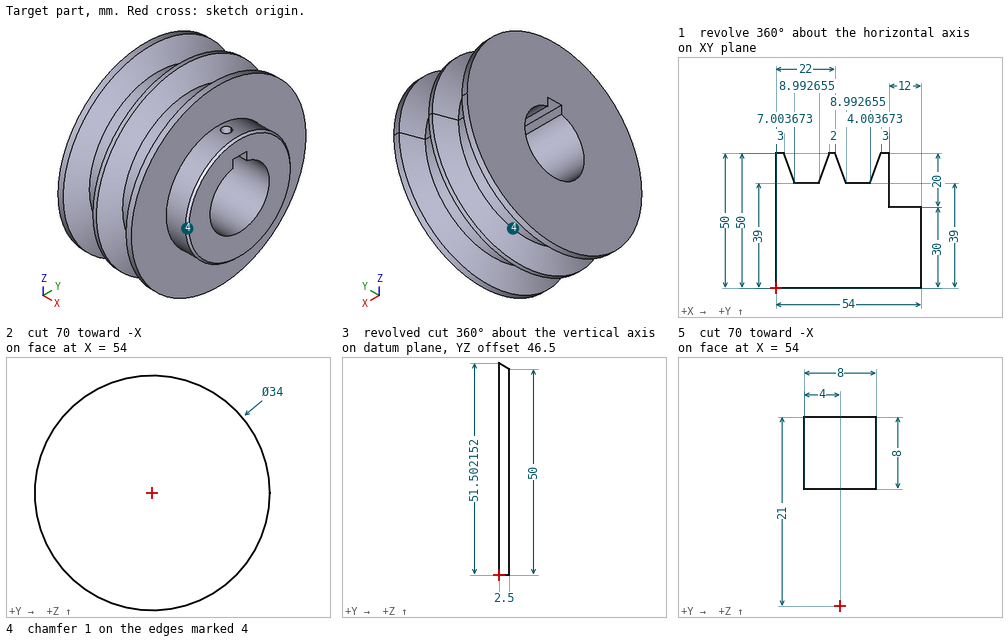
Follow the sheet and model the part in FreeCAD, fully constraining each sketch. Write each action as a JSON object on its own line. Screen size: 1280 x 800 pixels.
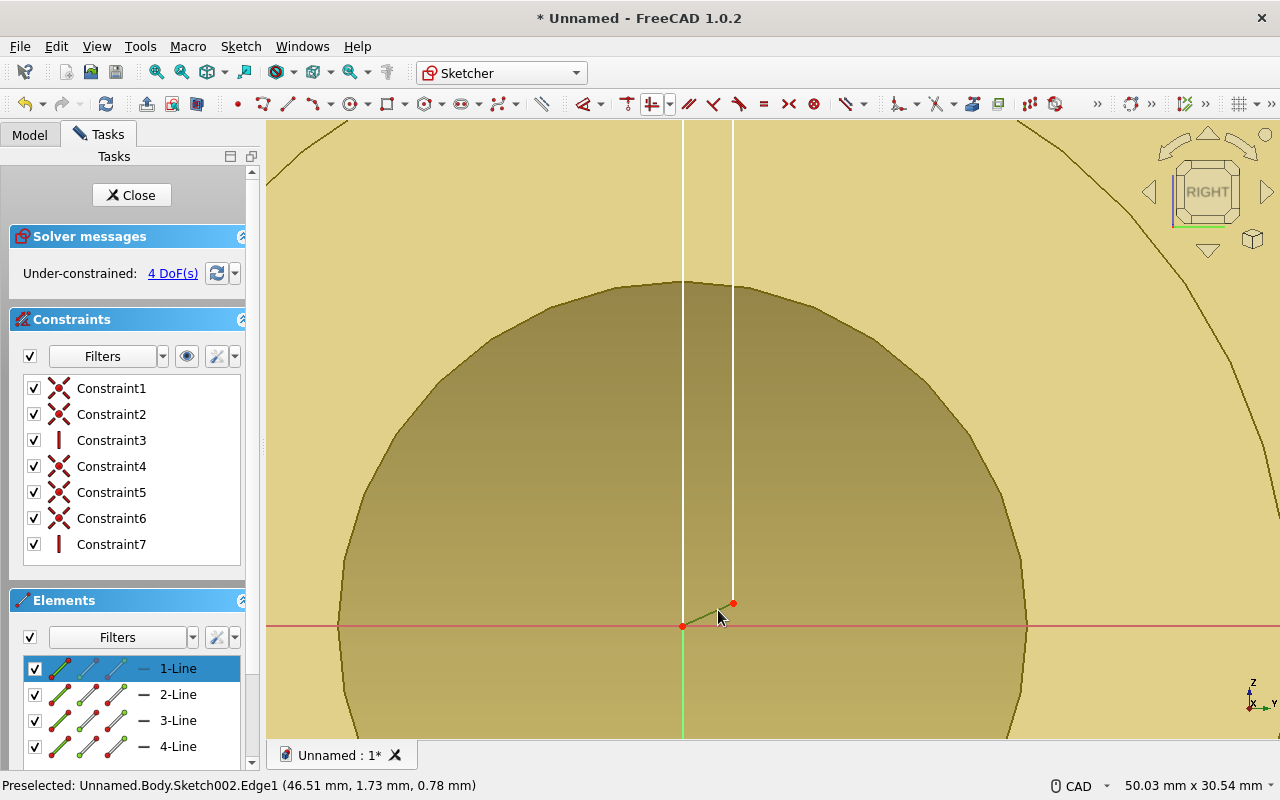
{"action": "key", "text": "h"}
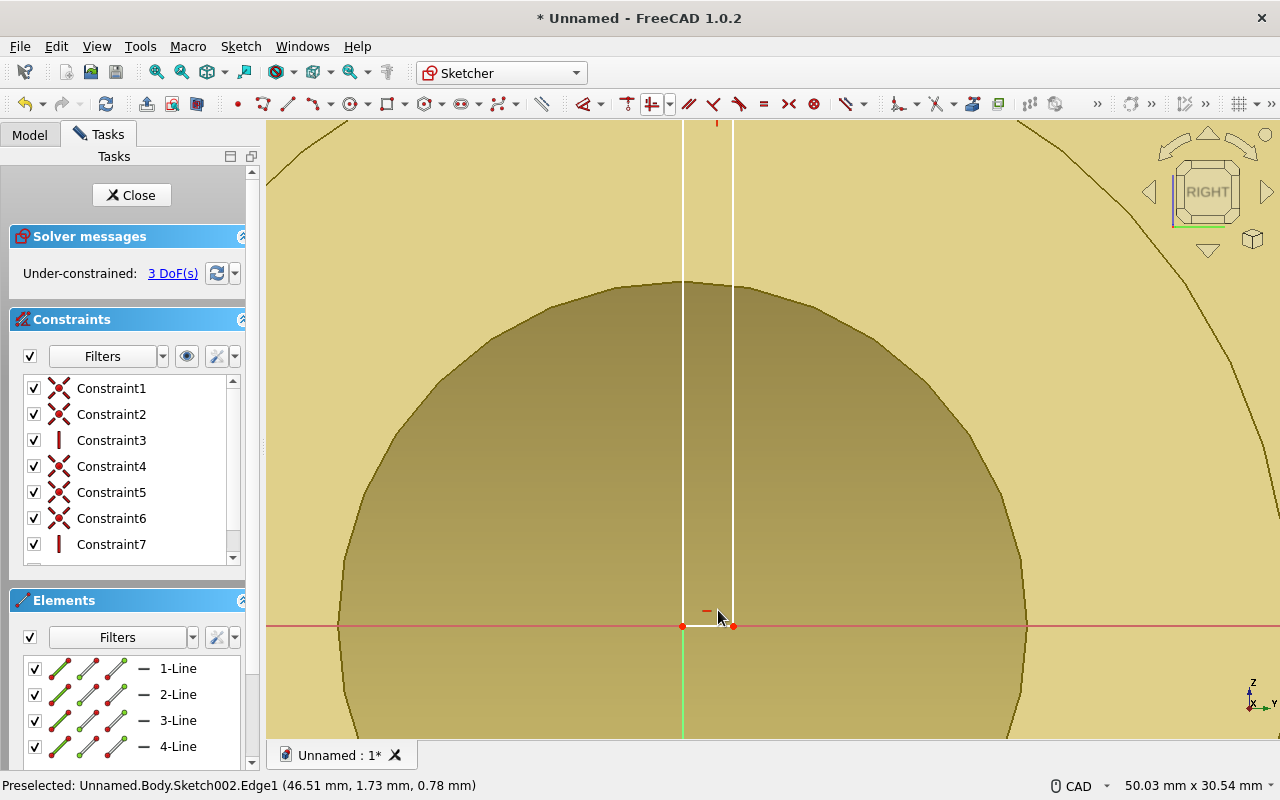
{"action": "key", "text": "d"}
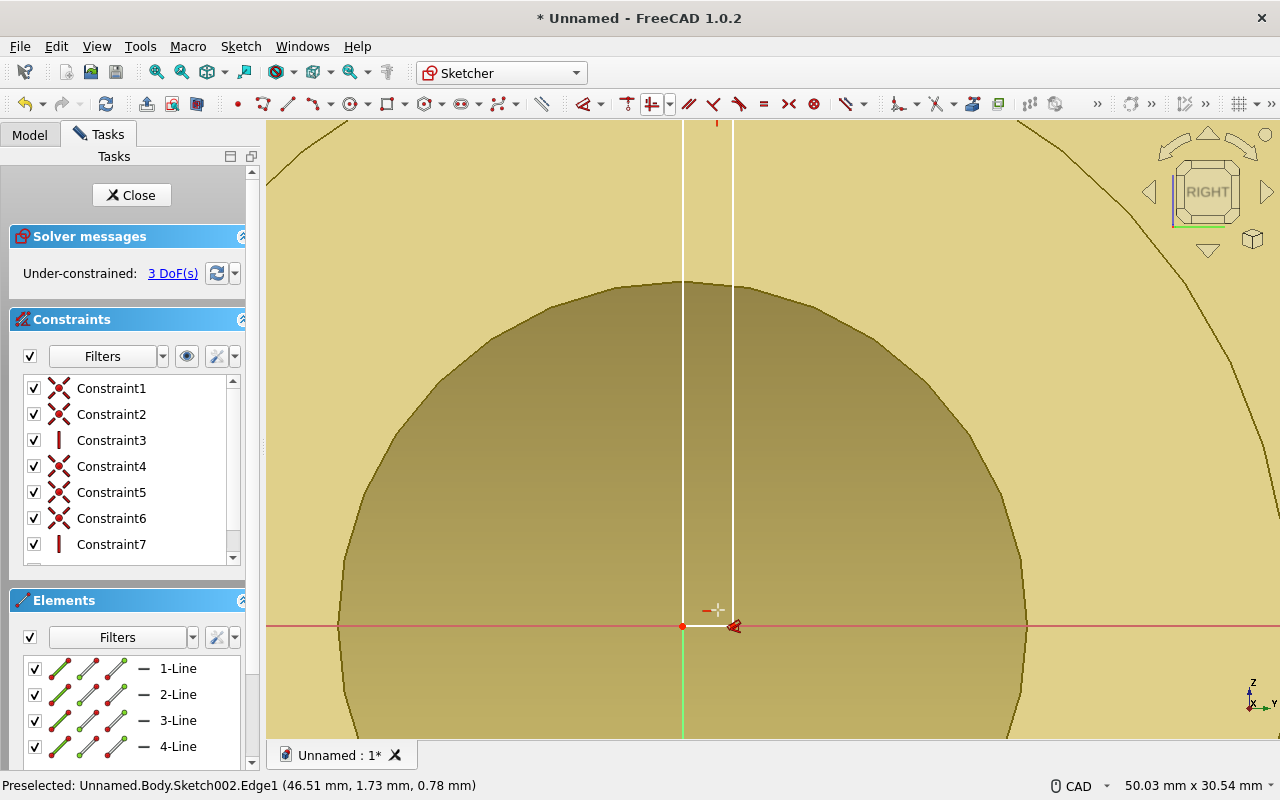
{"action": "left_click", "coordinate": [733, 323]}
{"action": "left_click", "coordinate": [767, 387]}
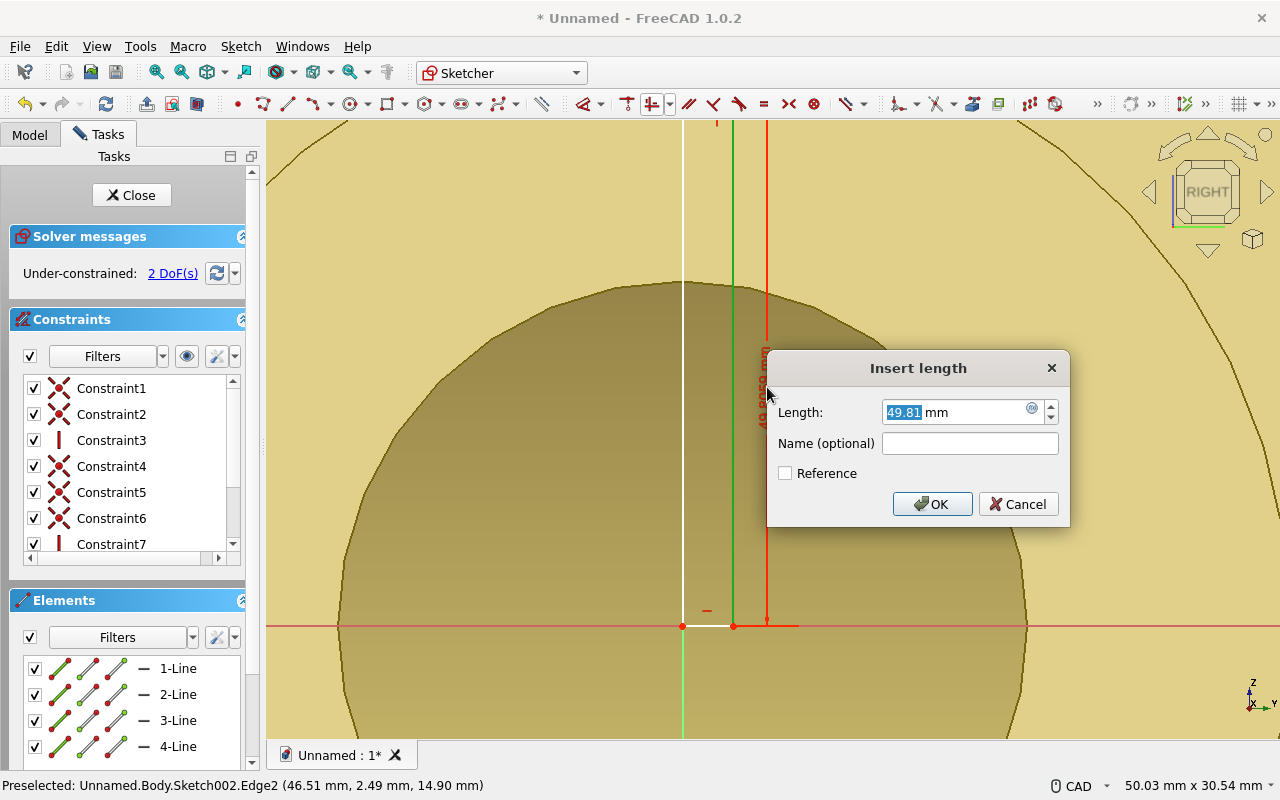
{"action": "type", "text": "50"}
{"action": "key", "text": "Return"}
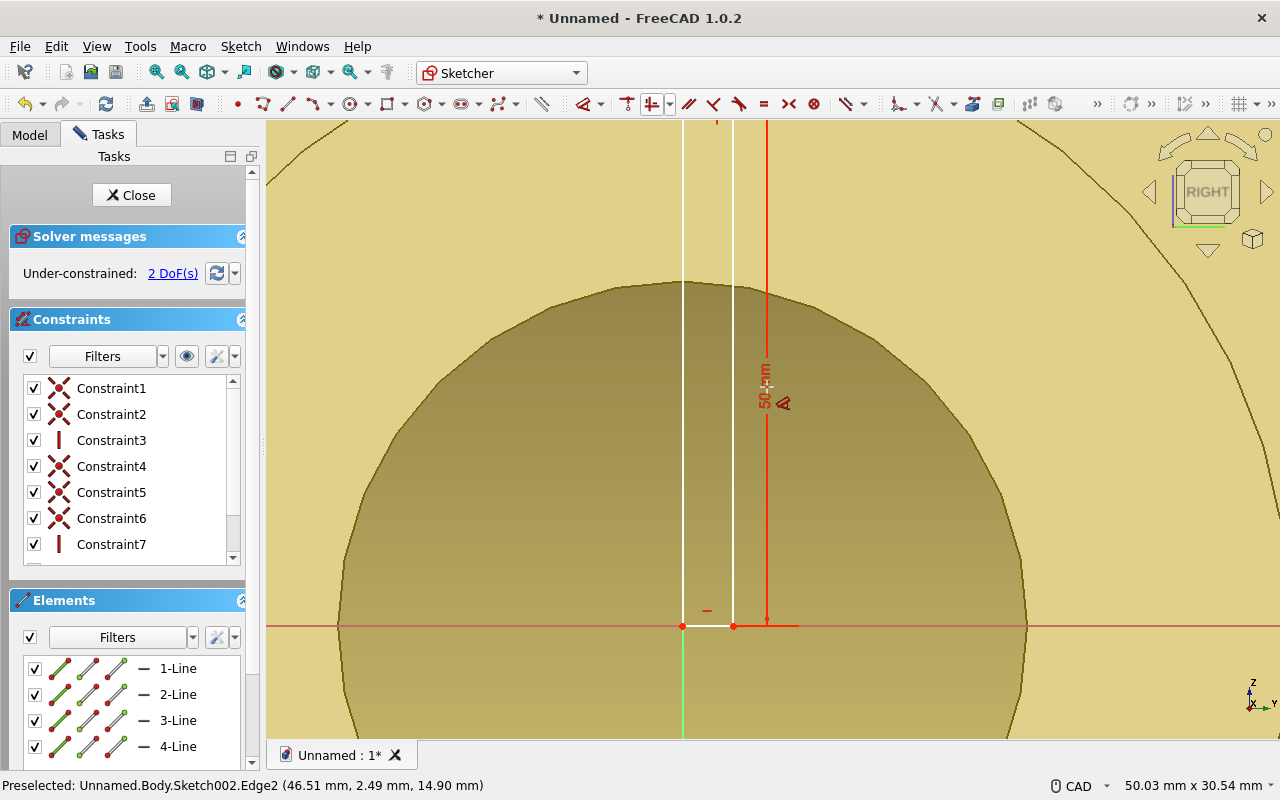
{"action": "left_click", "coordinate": [698, 626]}
{"action": "left_click", "coordinate": [708, 660]}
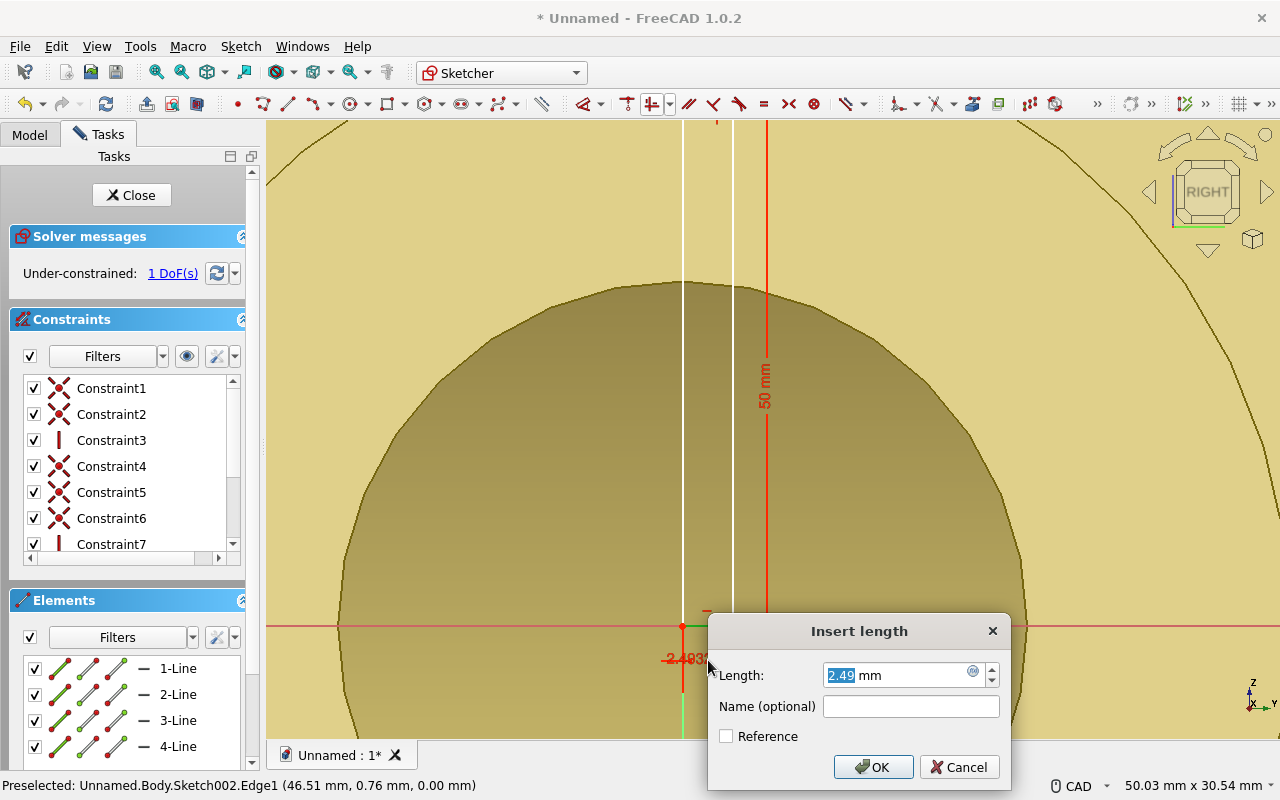
{"action": "type", "text": "2.5"}
{"action": "key", "text": "Return"}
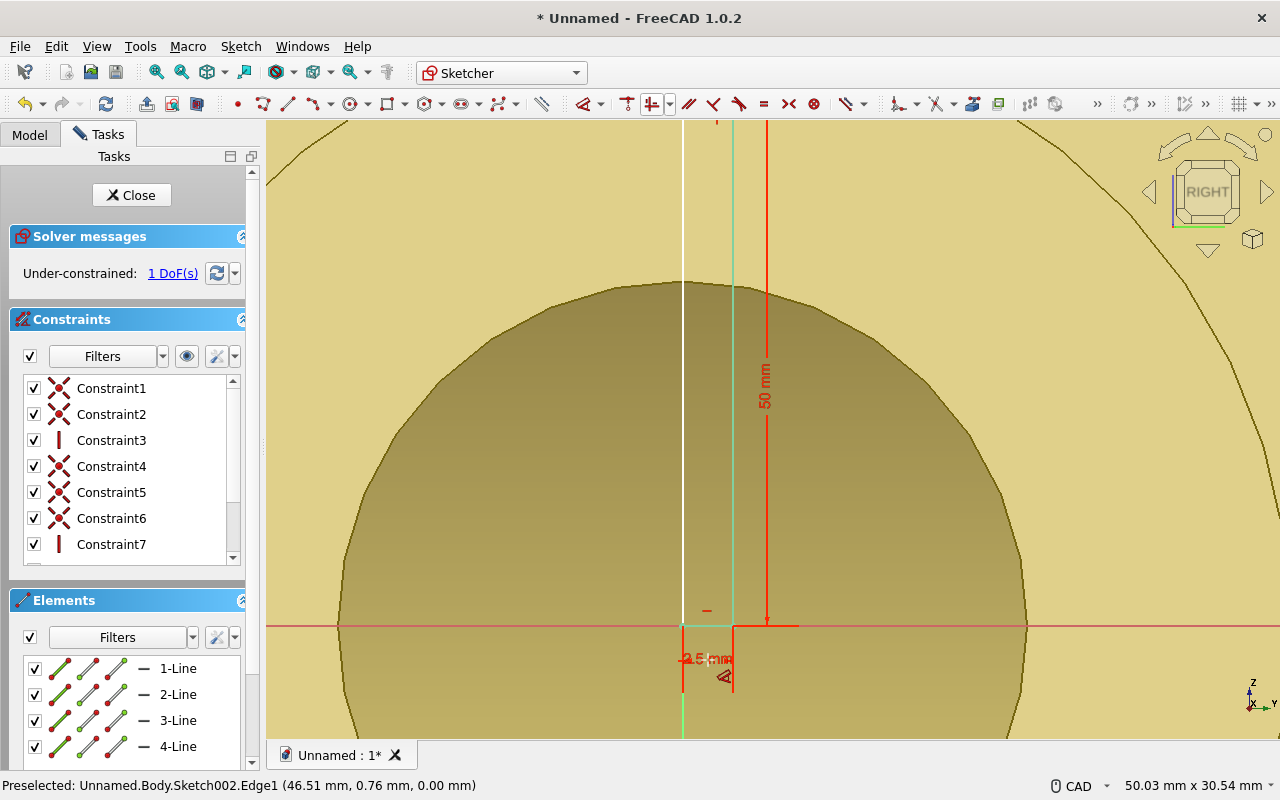
{"action": "left_click", "coordinate": [683, 313]}
{"action": "left_click", "coordinate": [649, 387]}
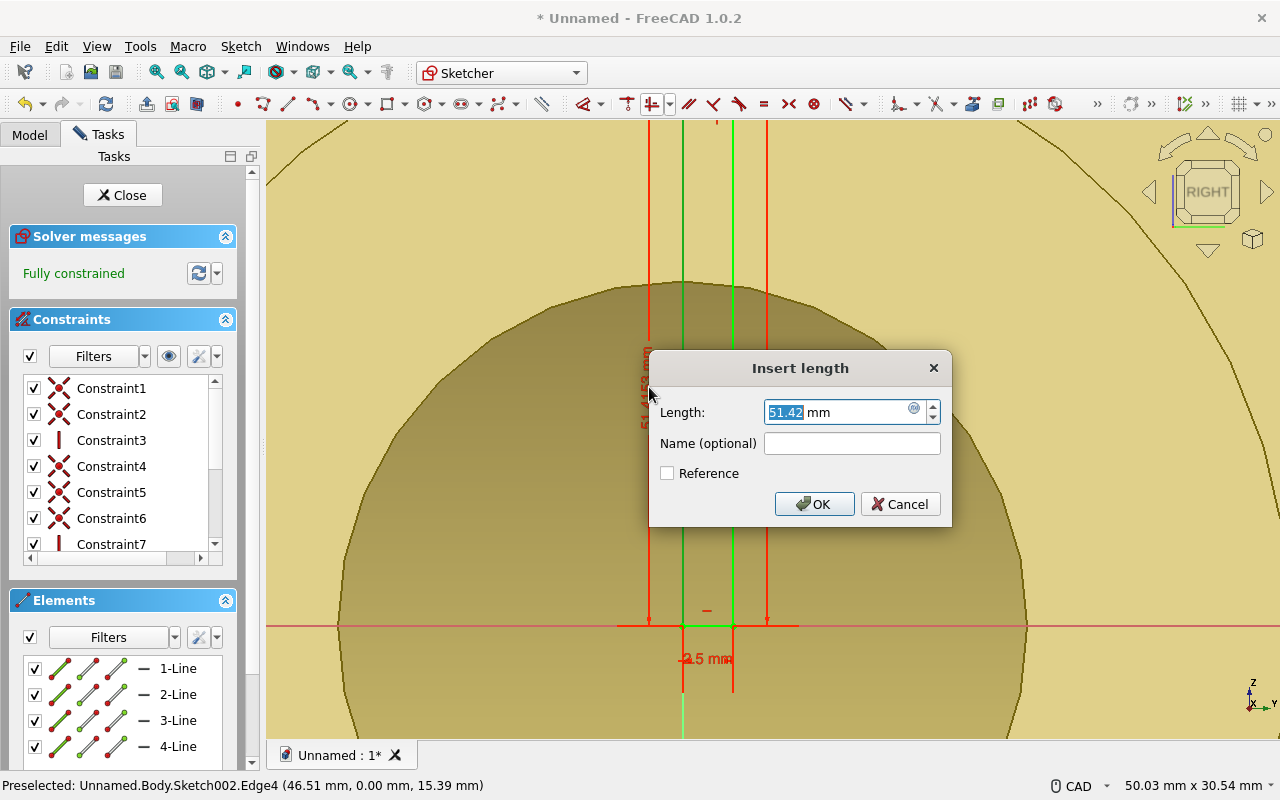
{"action": "type", "text": "51.502152"}
{"action": "key", "text": "Return"}
{"action": "key", "text": "Escape"}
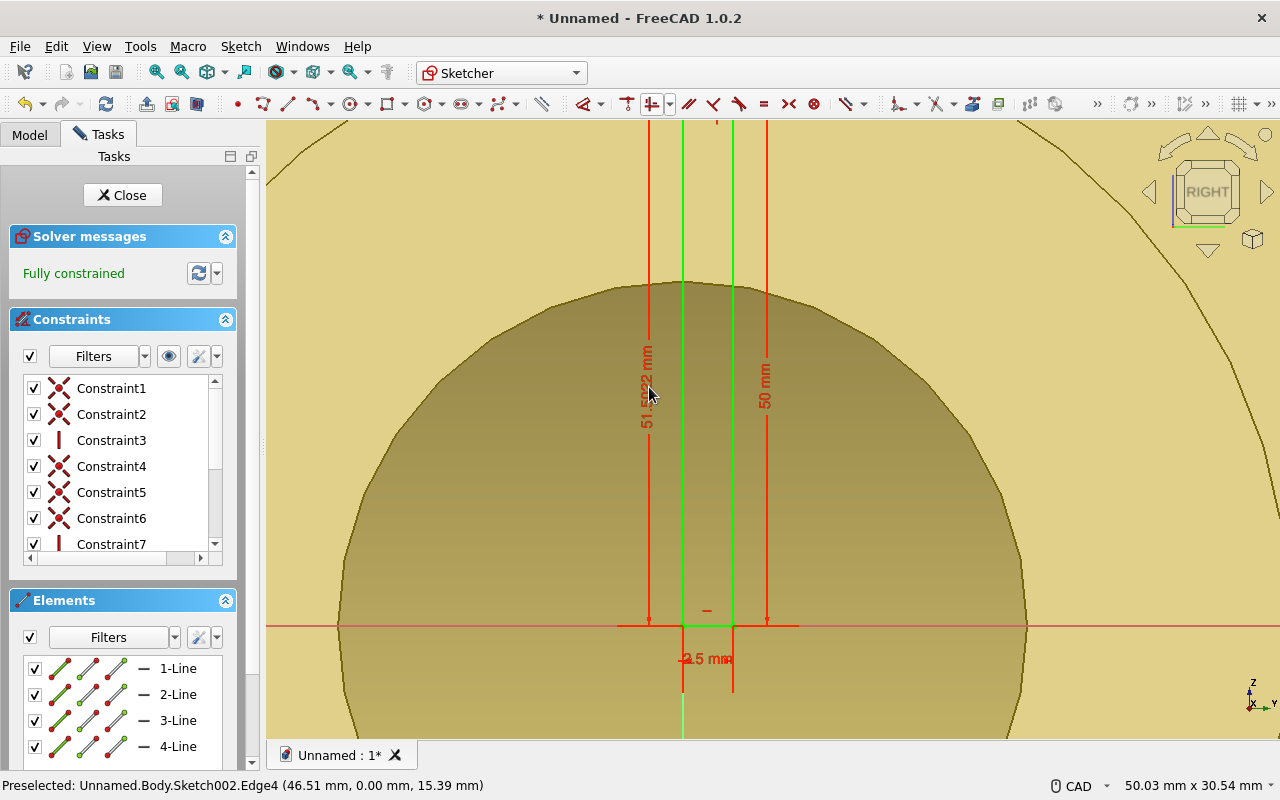
{"action": "left_click", "coordinate": [123, 195]}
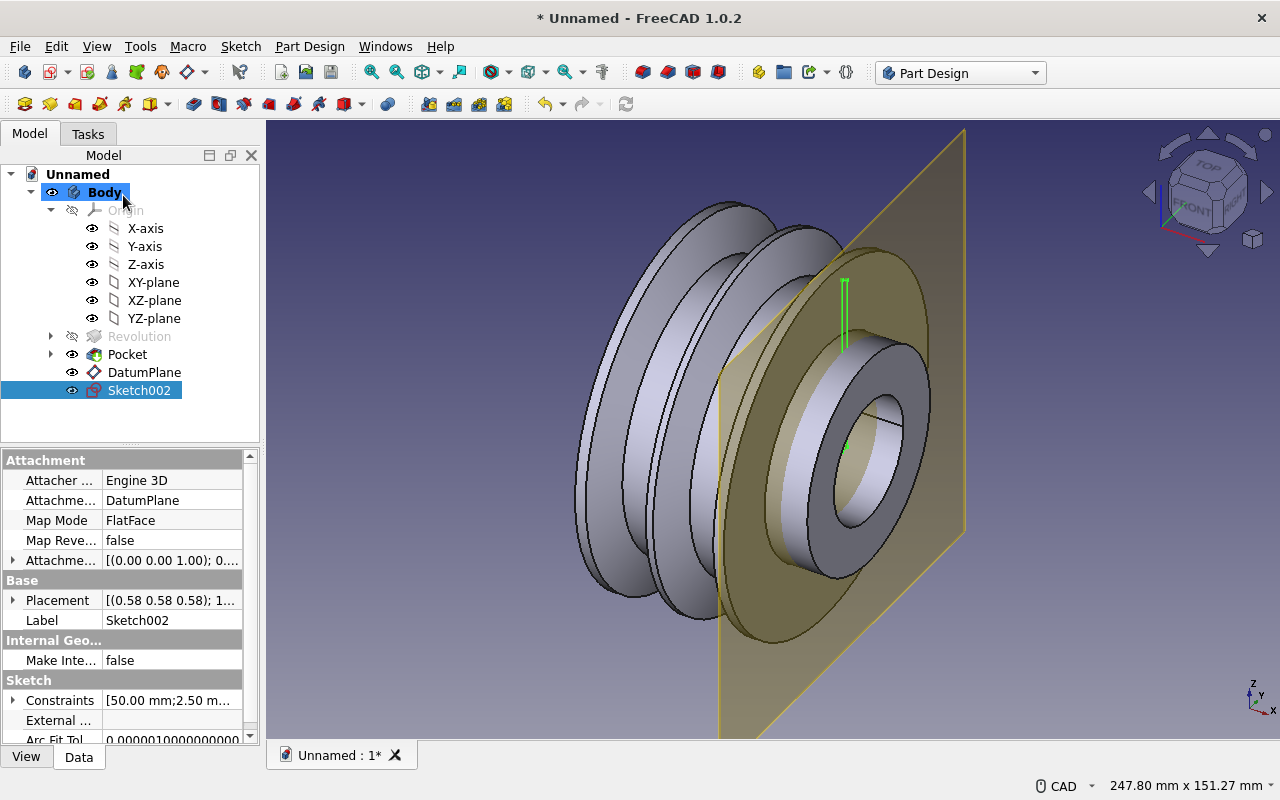
{"action": "left_click", "coordinate": [244, 104]}